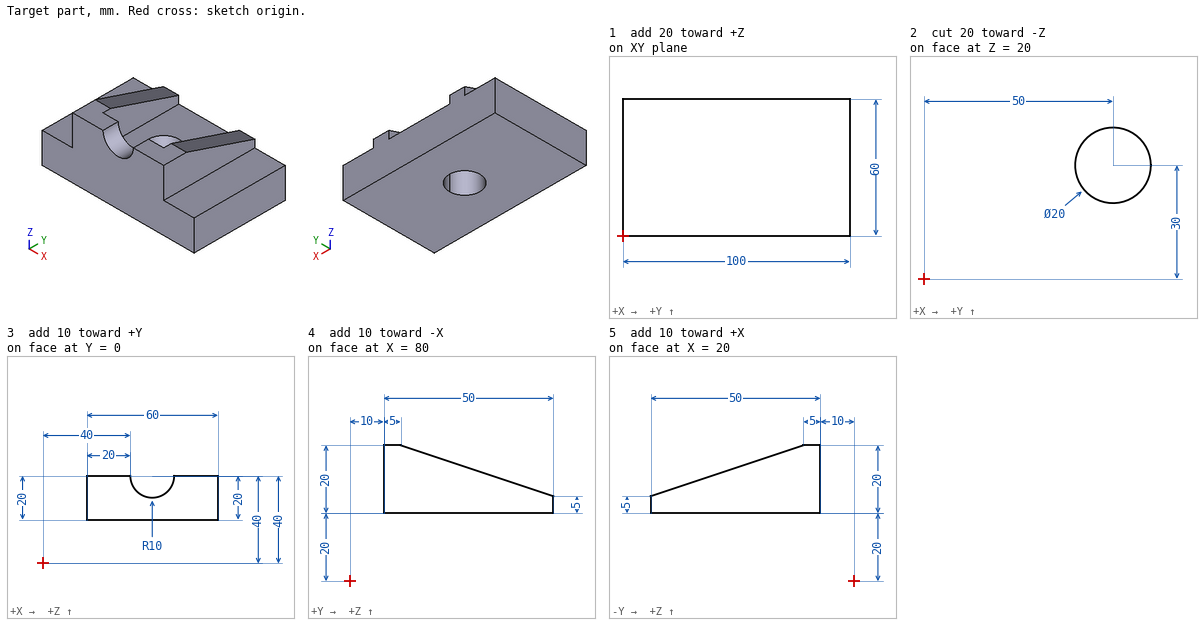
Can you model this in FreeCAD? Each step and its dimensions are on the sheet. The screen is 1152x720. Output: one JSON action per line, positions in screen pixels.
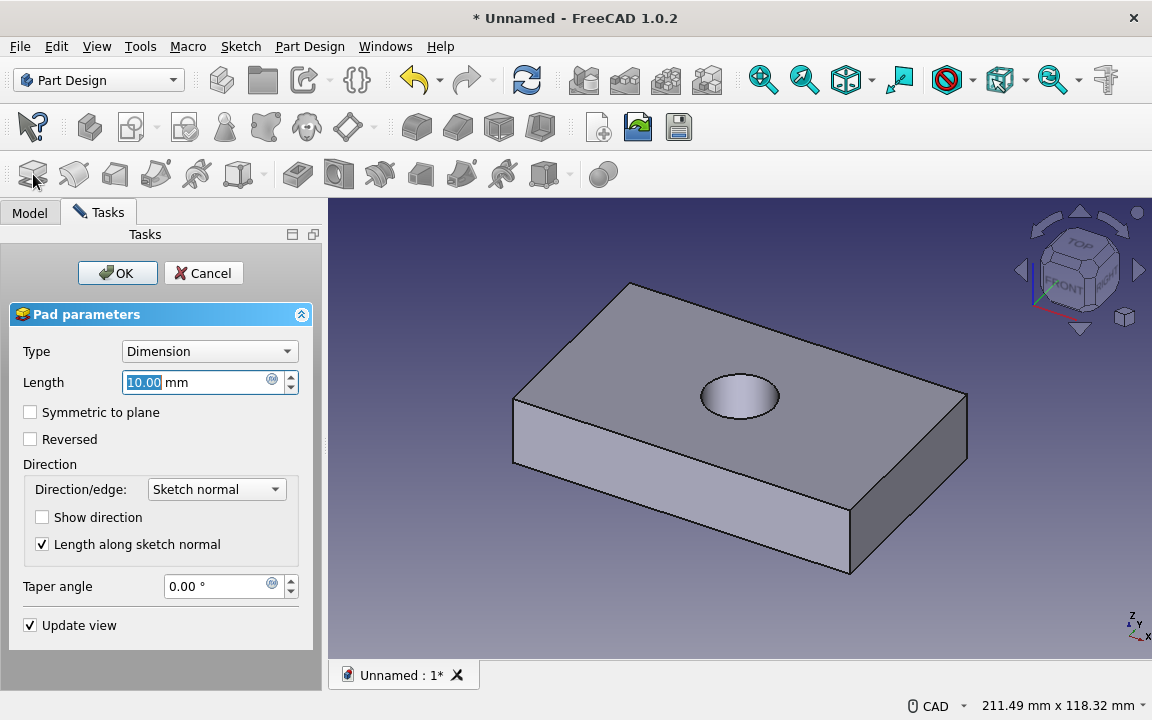
{"action": "type", "text": "10"}
{"action": "key", "text": "Tab"}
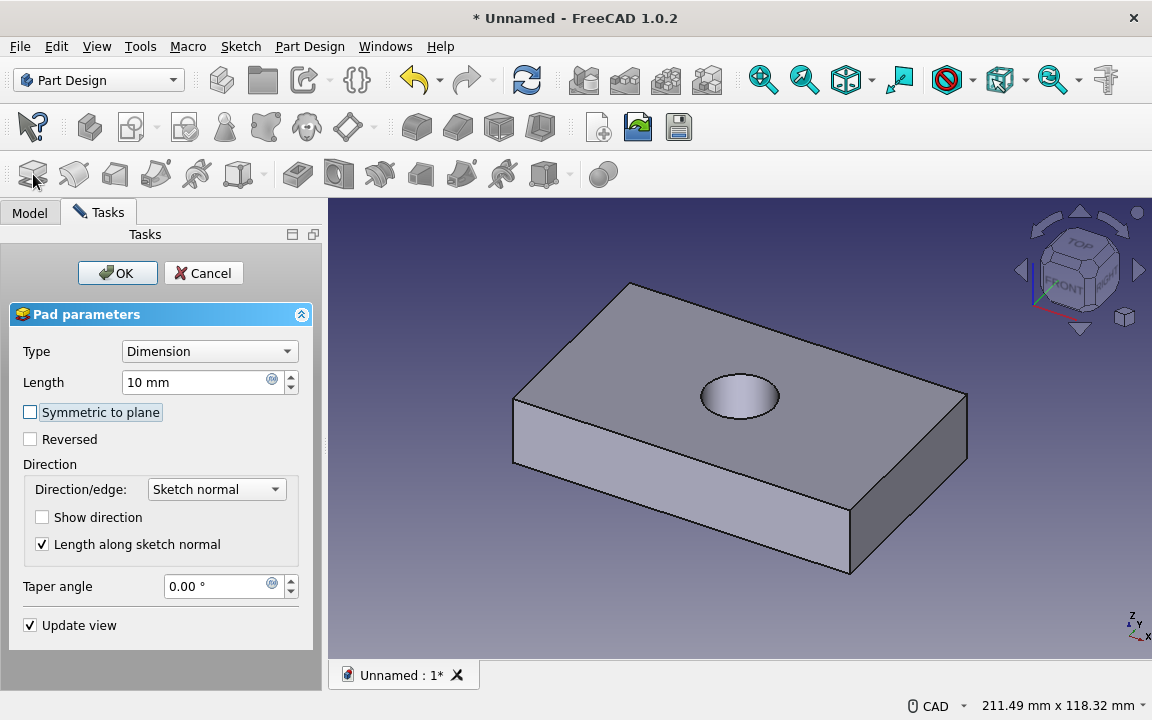
{"action": "left_click", "coordinate": [31, 439]}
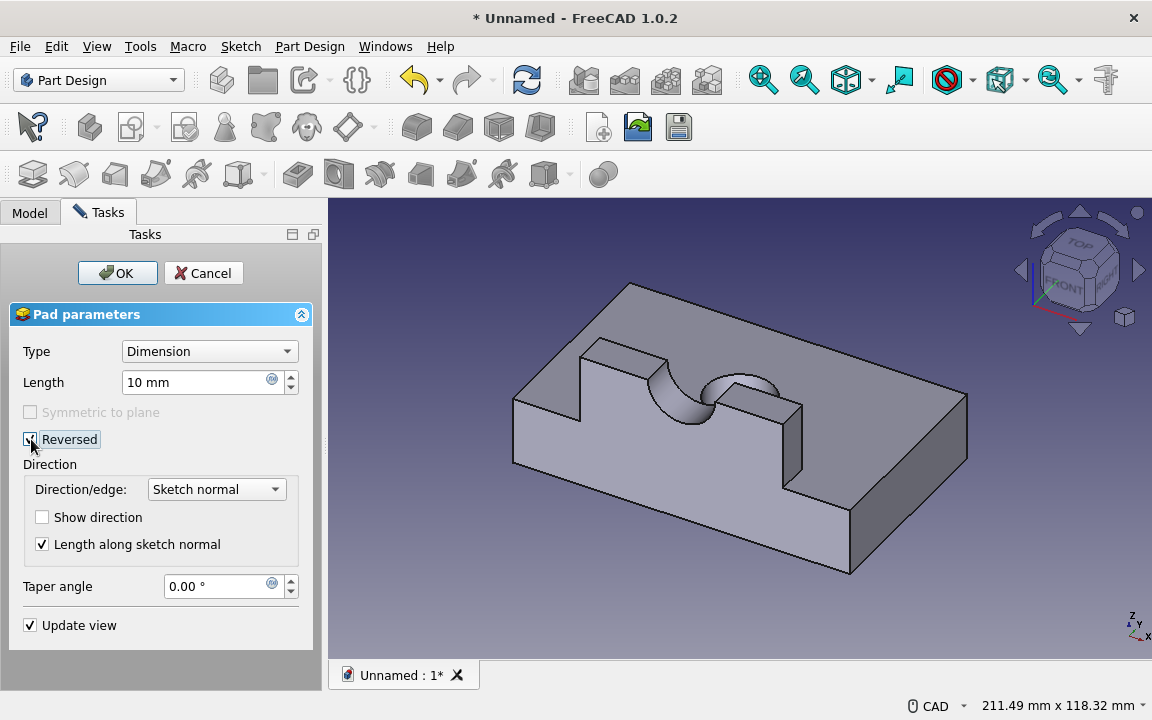
{"action": "left_click", "coordinate": [118, 273]}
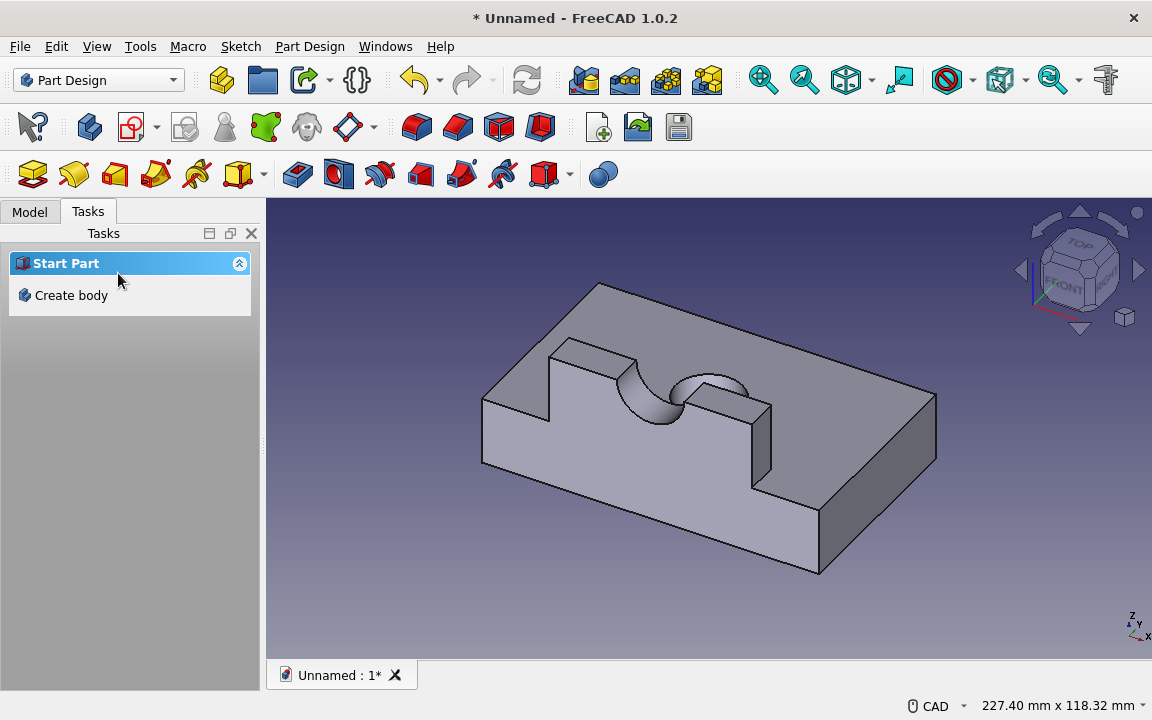
{"action": "left_click", "coordinate": [762, 436]}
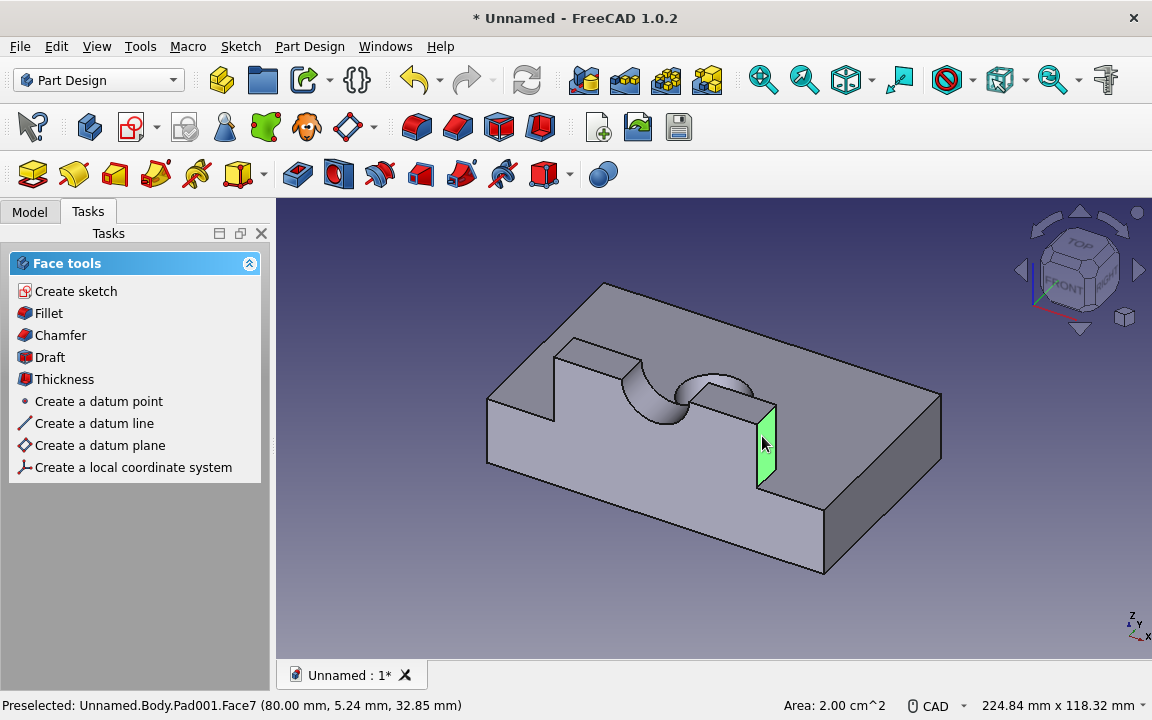
{"action": "left_click", "coordinate": [130, 128]}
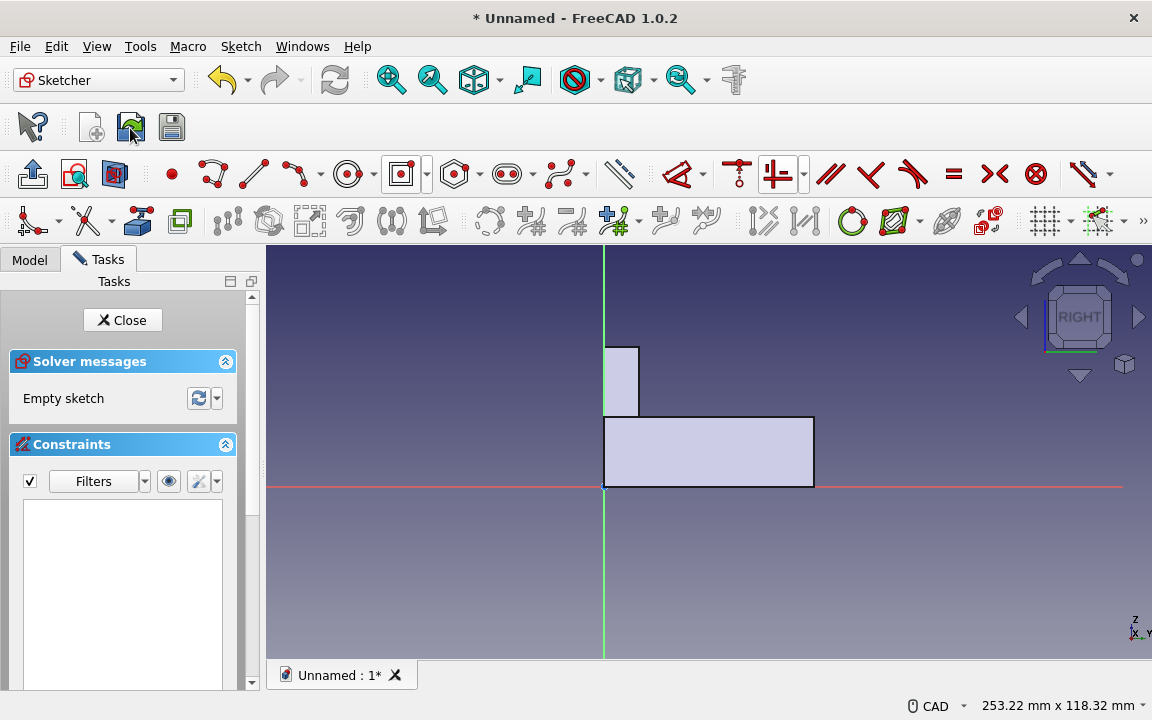
{"action": "scroll", "coordinate": [792, 374], "scroll_direction": "up", "scroll_amount": 3}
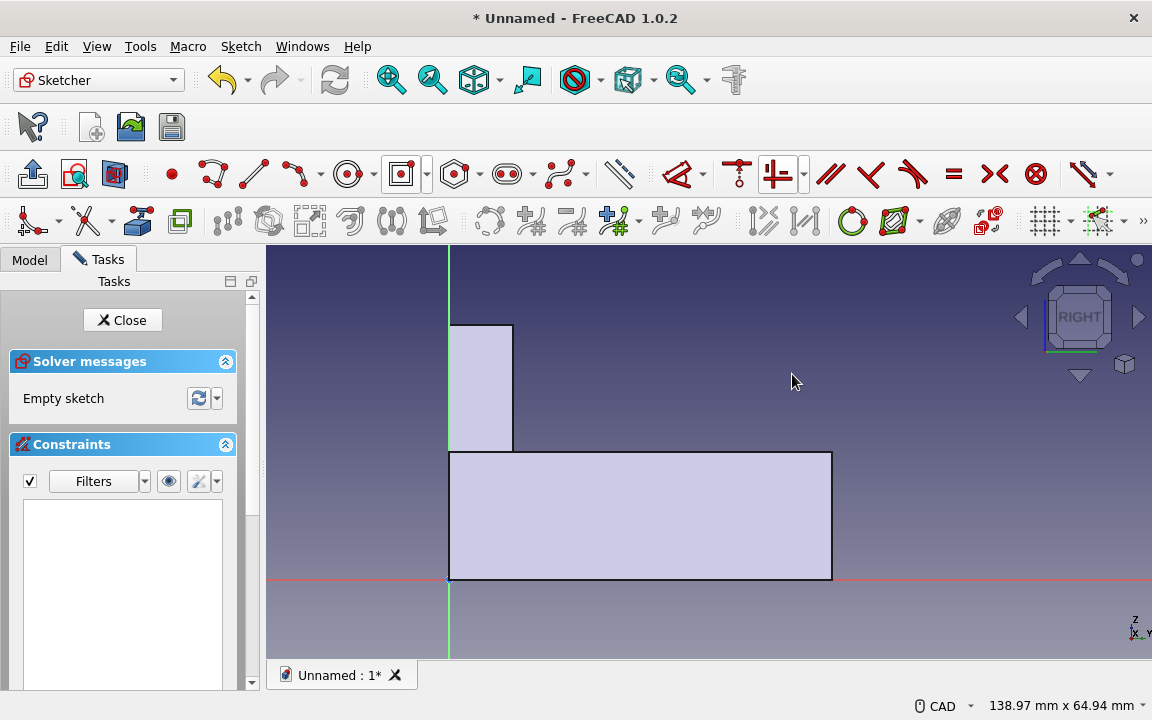
{"action": "left_click", "coordinate": [213, 174]}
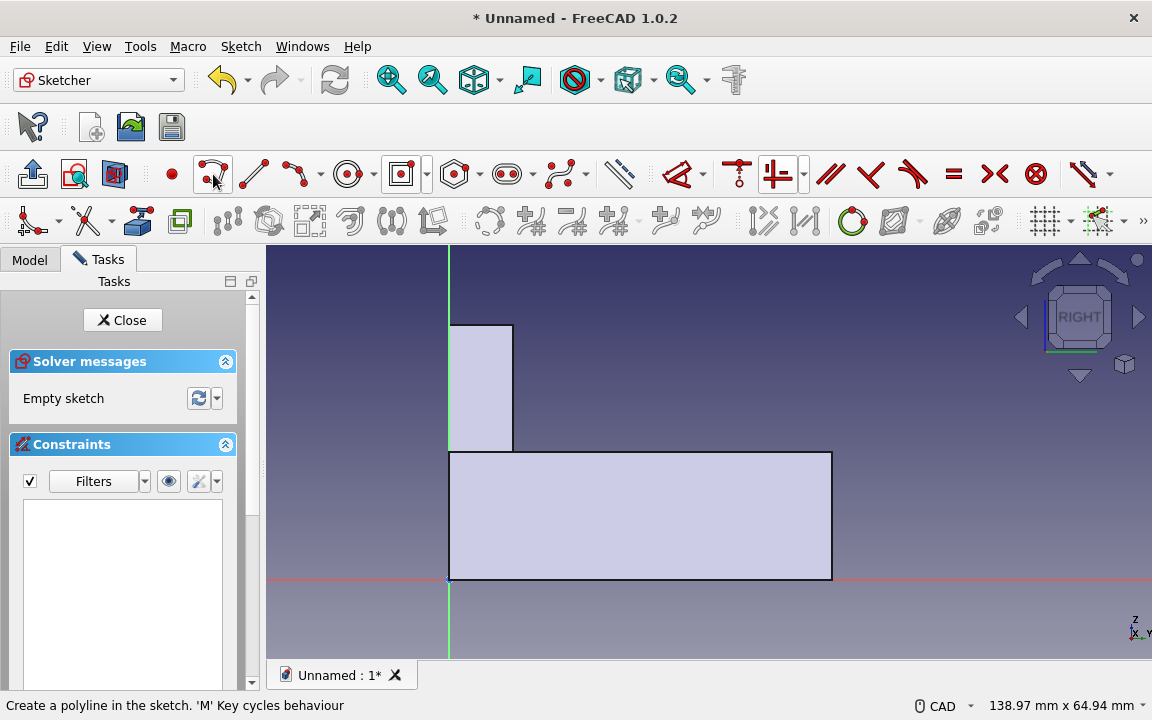
{"action": "left_click", "coordinate": [513, 452]}
{"action": "left_click", "coordinate": [832, 452]}
{"action": "left_click", "coordinate": [832, 420]}
{"action": "left_click", "coordinate": [545, 325]}
{"action": "left_click", "coordinate": [513, 325]}
{"action": "left_click", "coordinate": [513, 453]}
{"action": "key", "text": "Escape"}
{"action": "key", "text": "Escape"}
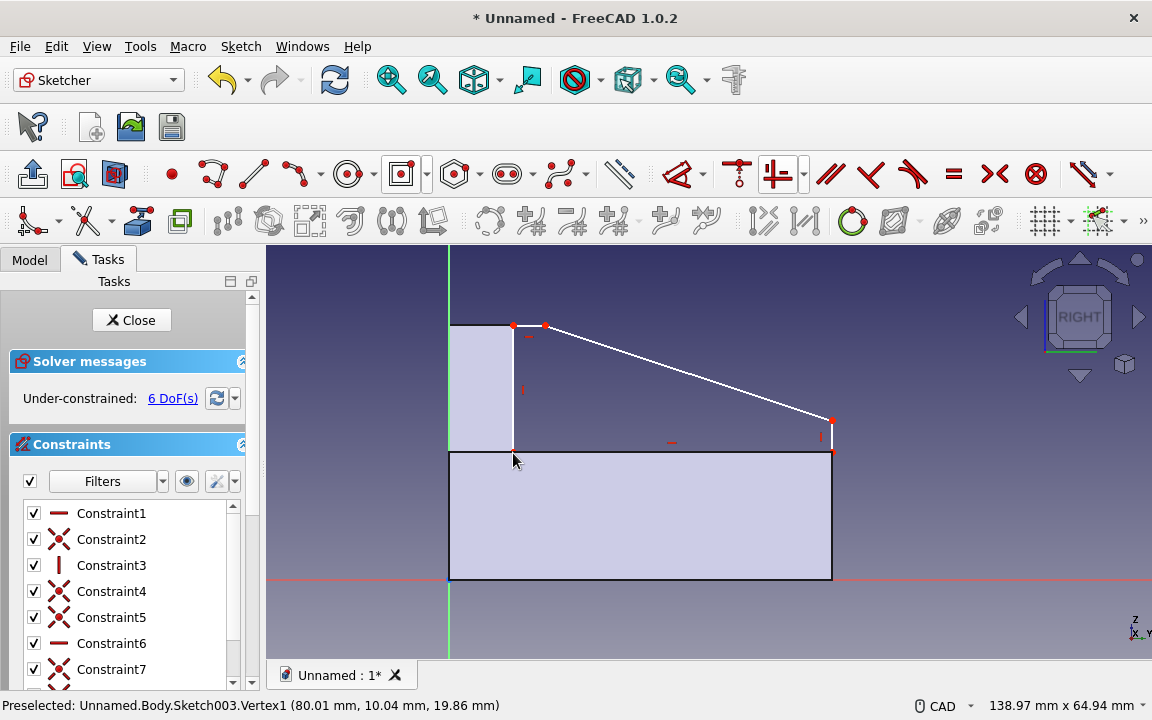
{"action": "left_click", "coordinate": [676, 174]}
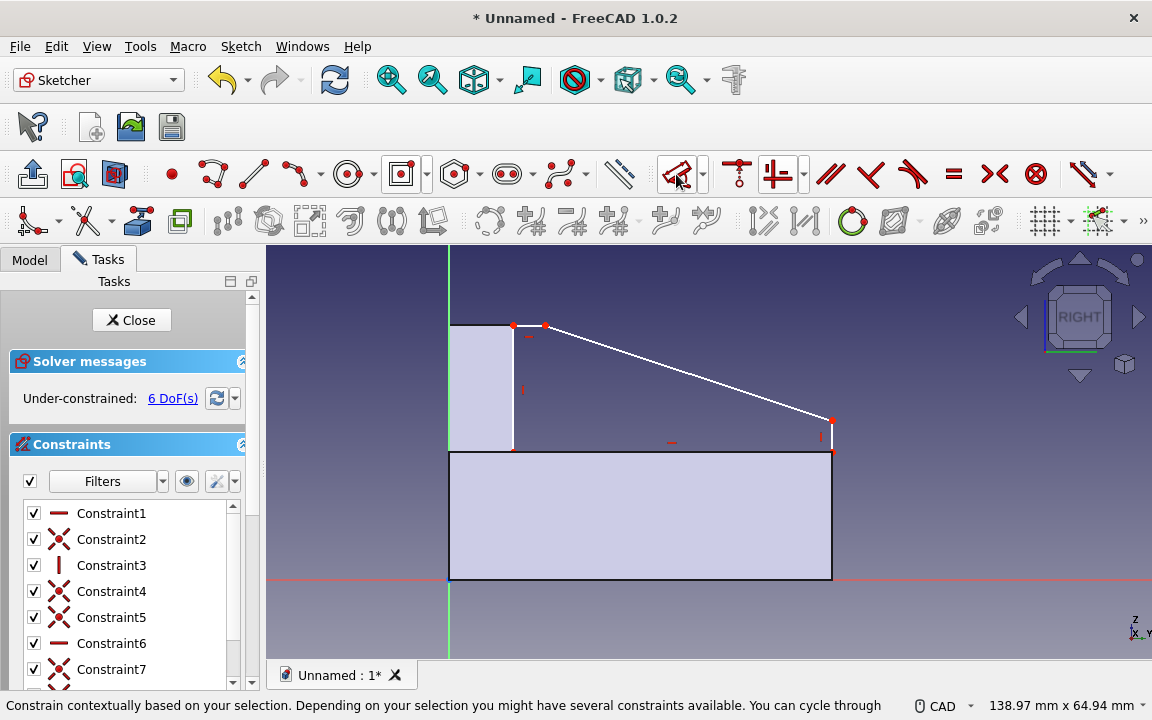
{"action": "scroll", "coordinate": [832, 443], "scroll_direction": "up", "scroll_amount": 2}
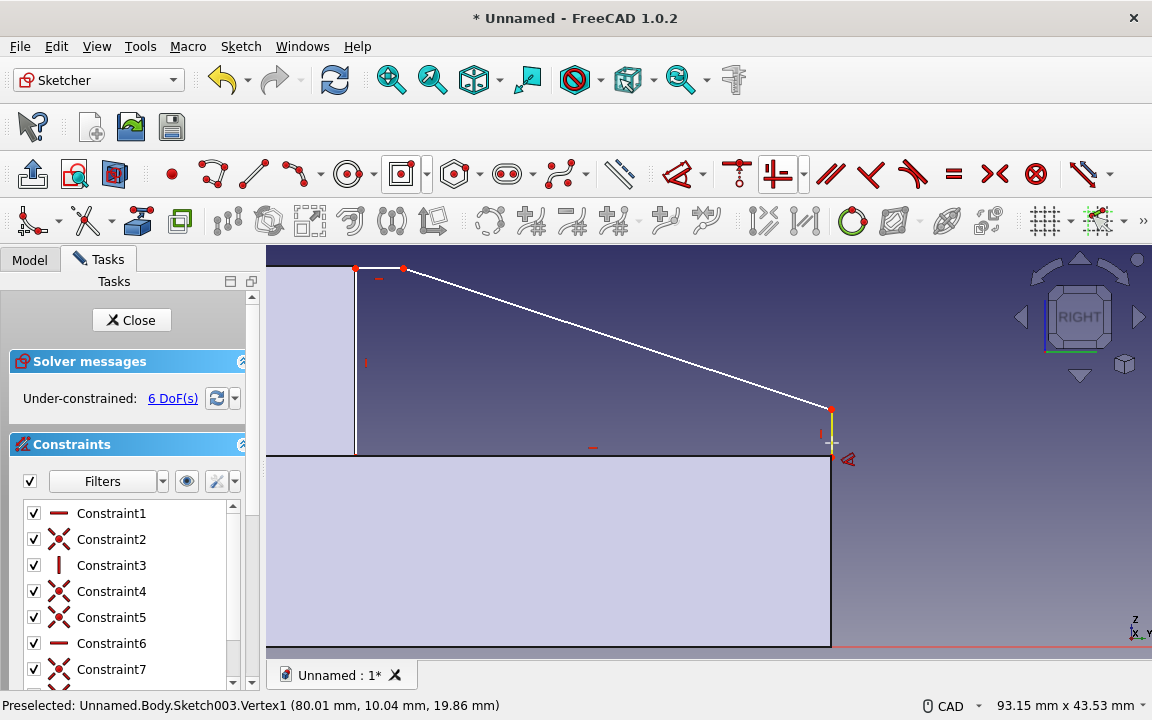
{"action": "left_click", "coordinate": [832, 443]}
{"action": "left_click", "coordinate": [866, 434]}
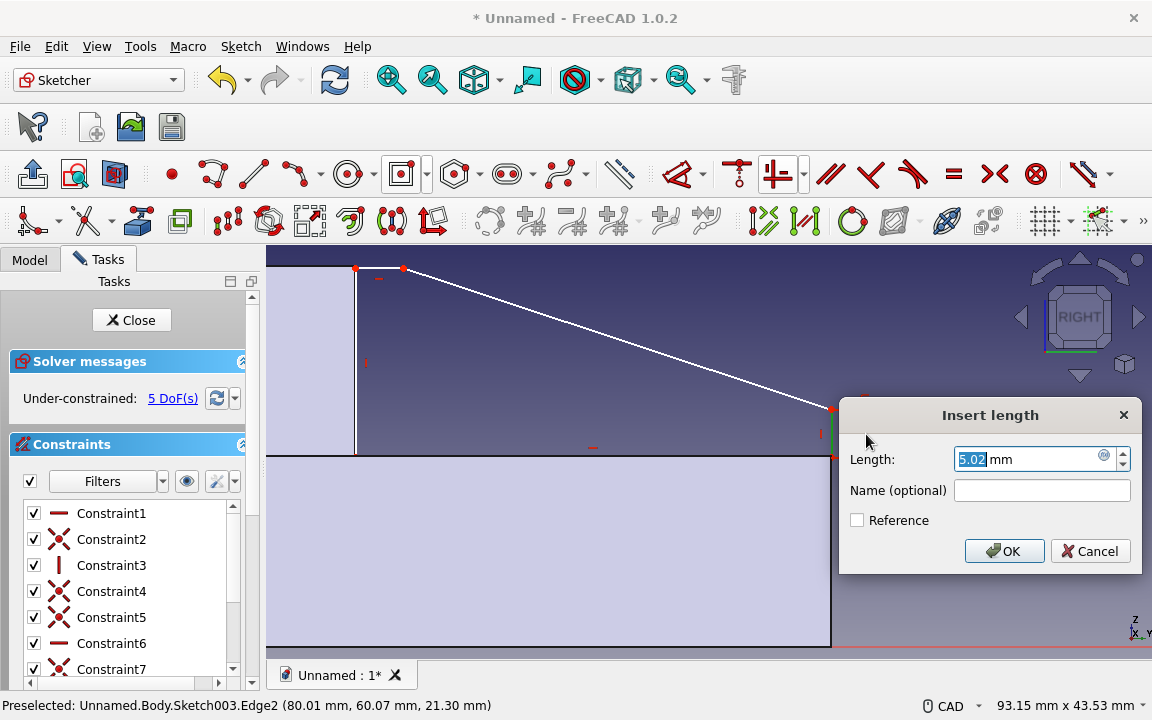
{"action": "type", "text": "5"}
{"action": "key", "text": "Return"}